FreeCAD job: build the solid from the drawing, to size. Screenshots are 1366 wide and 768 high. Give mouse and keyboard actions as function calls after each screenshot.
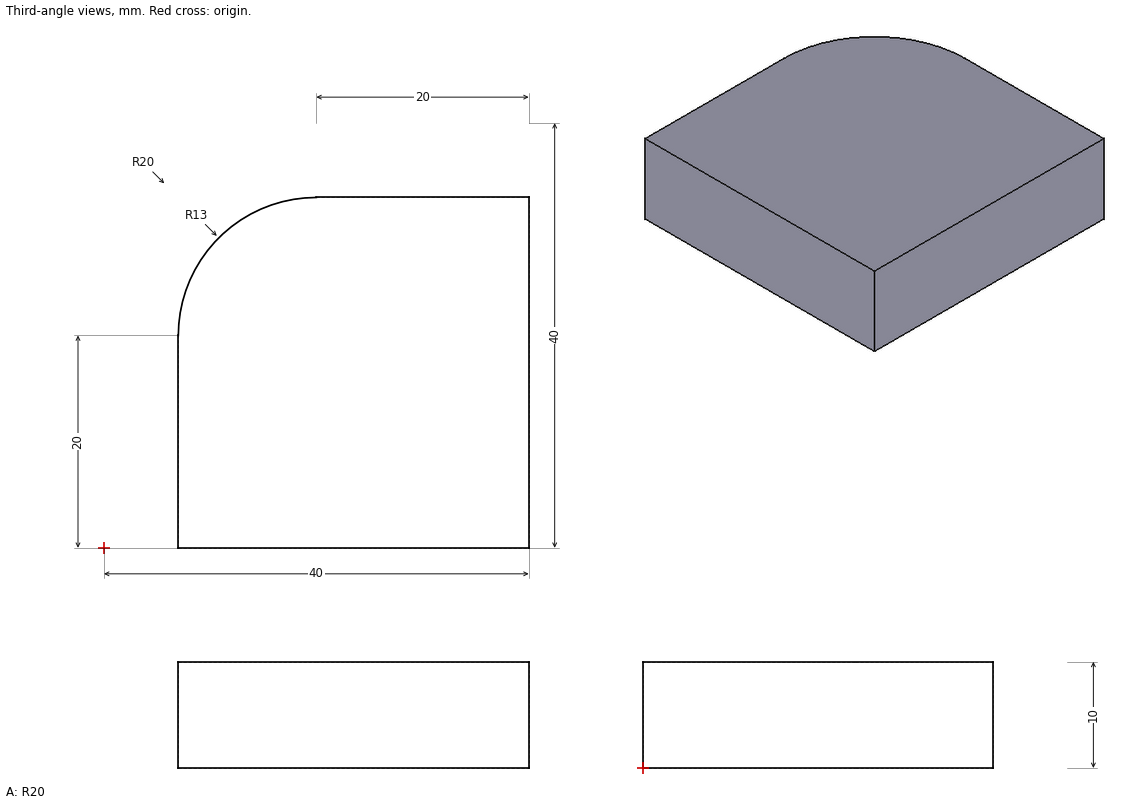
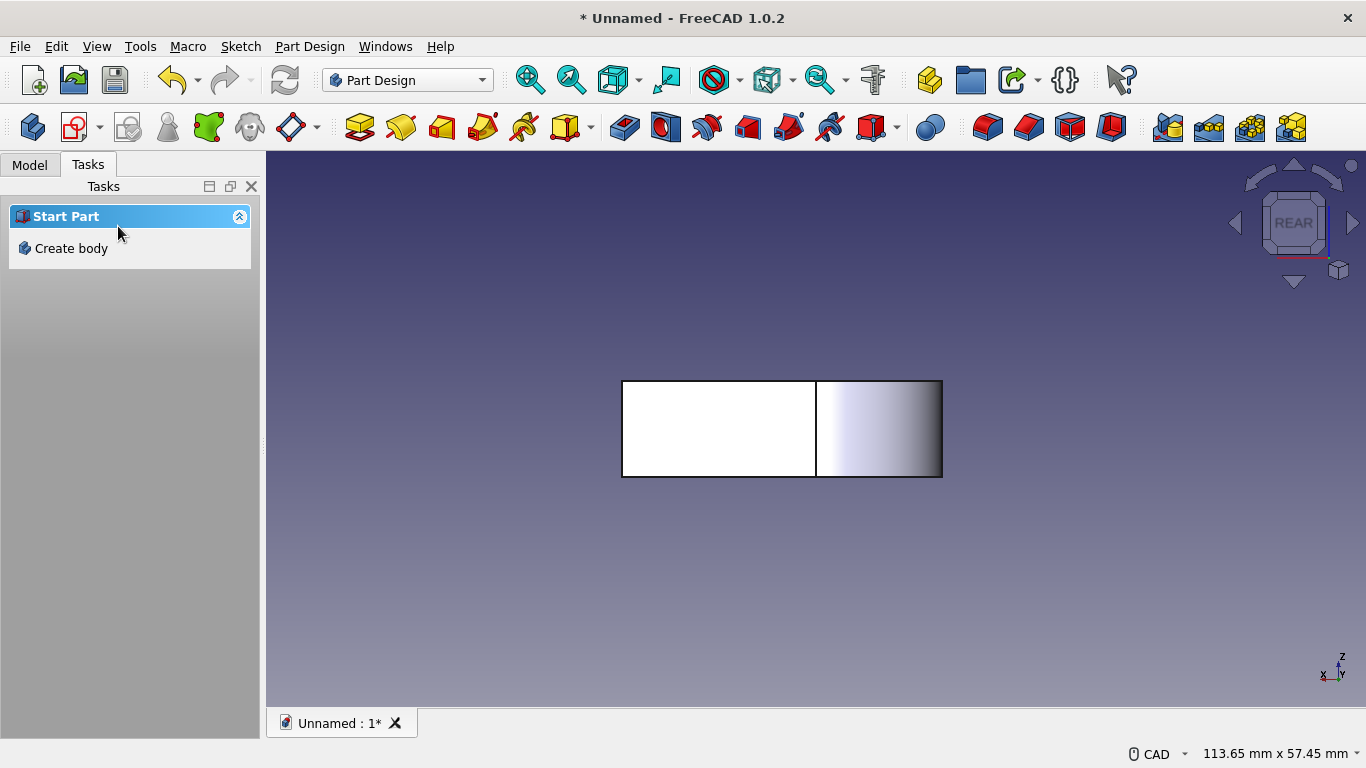
key(0)